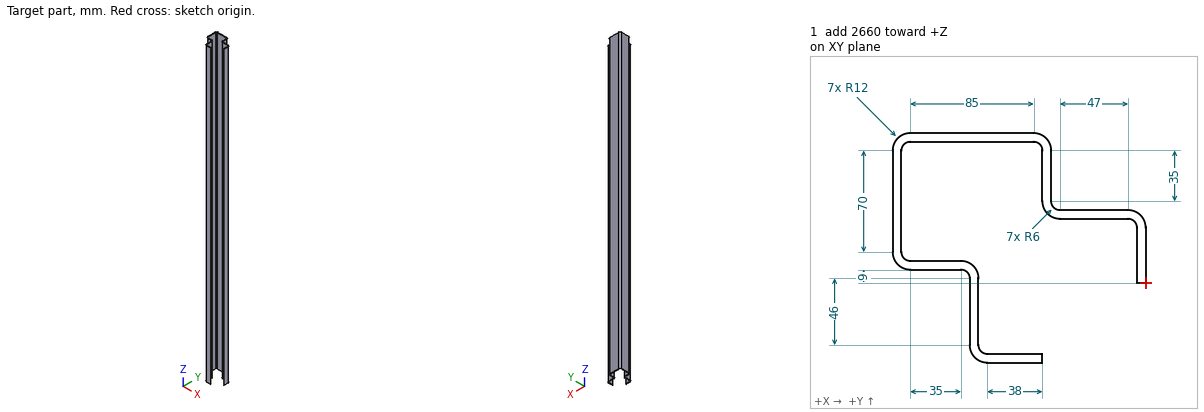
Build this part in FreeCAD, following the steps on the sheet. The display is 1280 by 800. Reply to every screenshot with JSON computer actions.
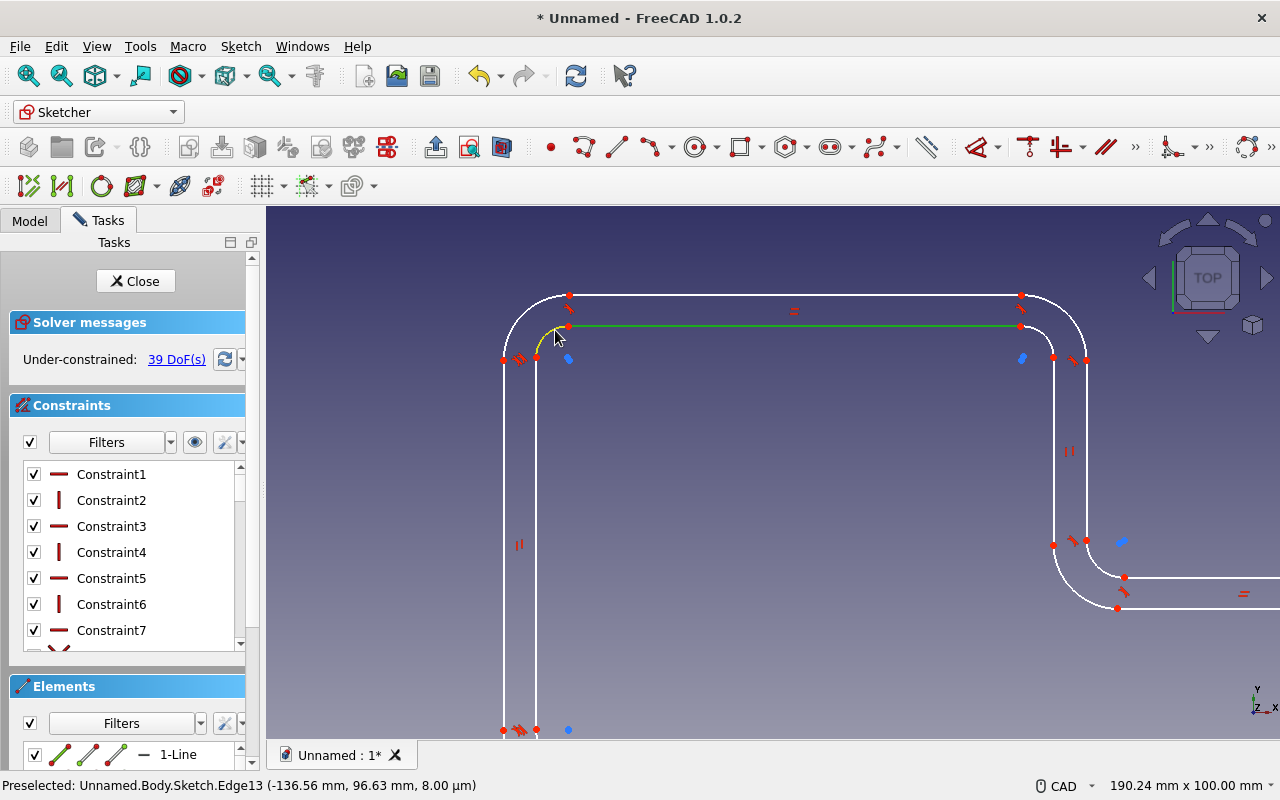
{"action": "left_click", "coordinate": [554, 329]}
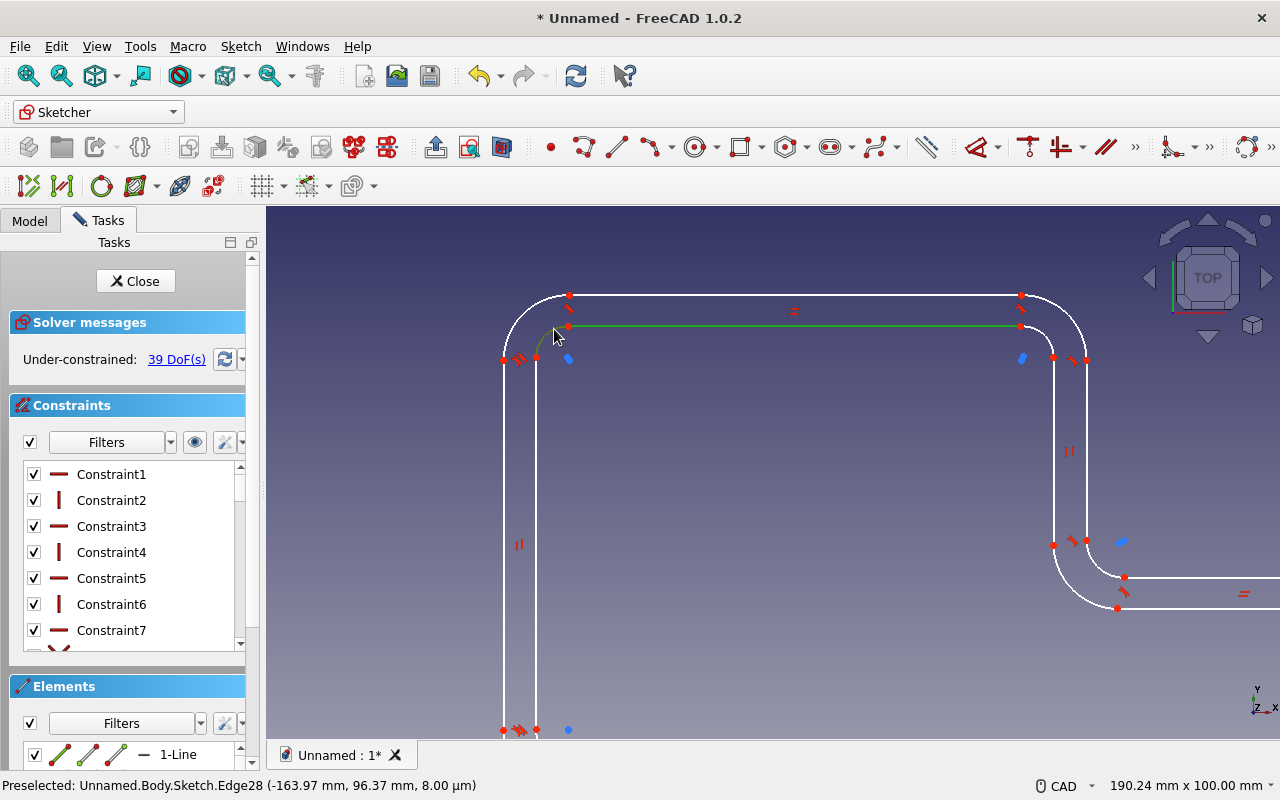
{"action": "key", "text": "t"}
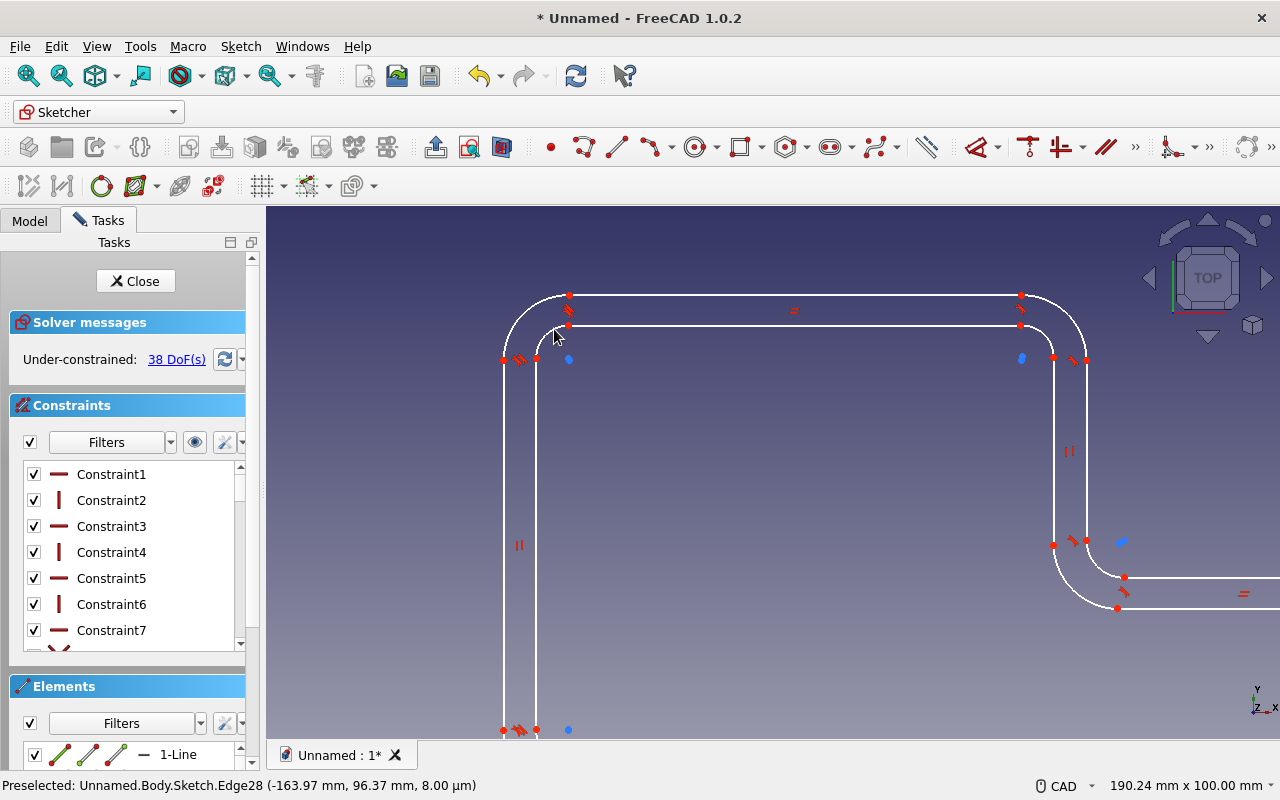
{"action": "left_click", "coordinate": [704, 326]}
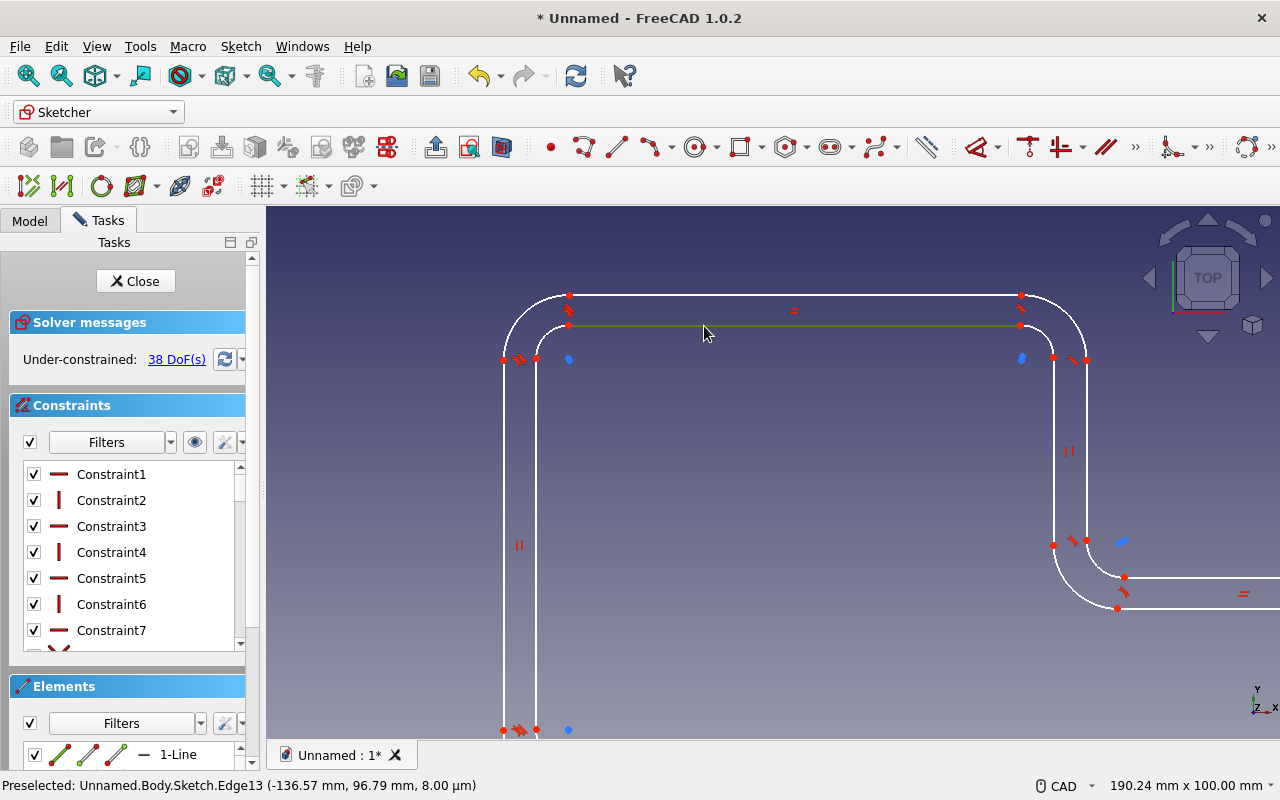
{"action": "left_click", "coordinate": [1050, 343]}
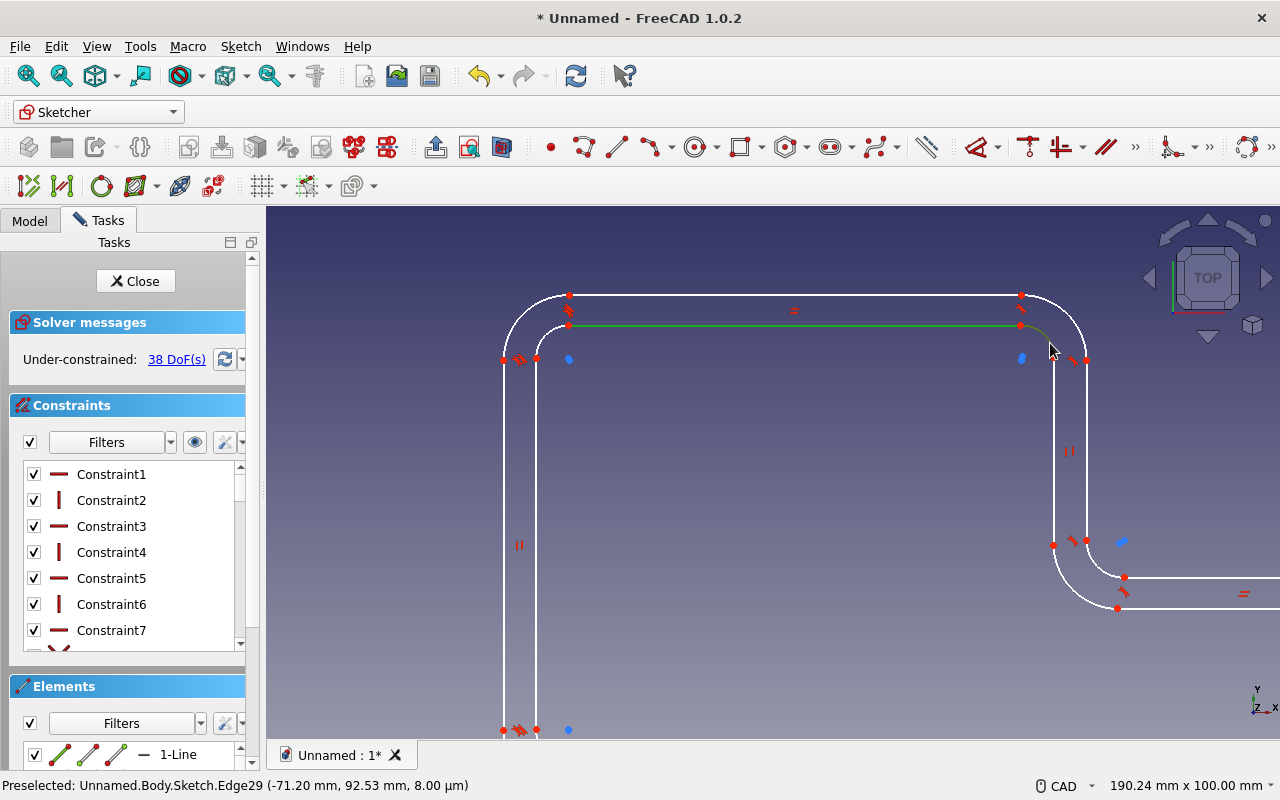
{"action": "key", "text": "t"}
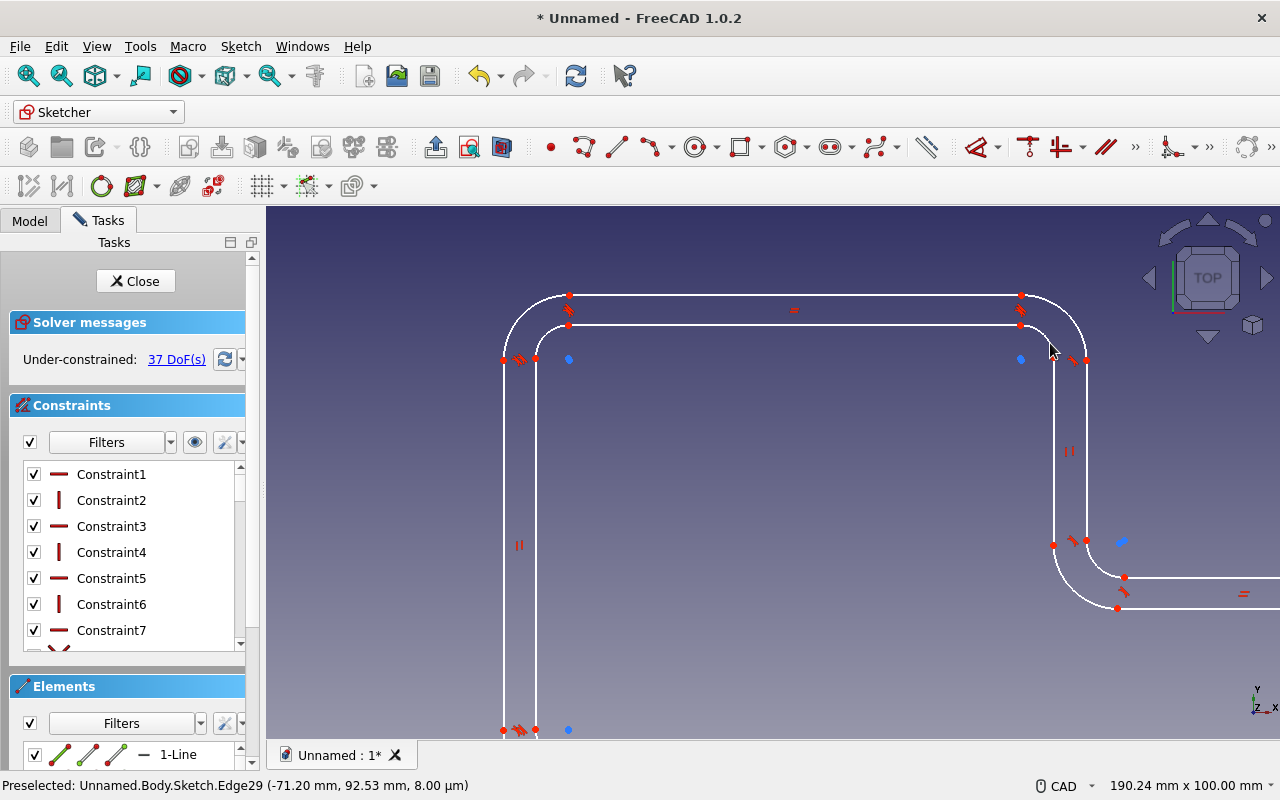
{"action": "left_click", "coordinate": [1054, 414]}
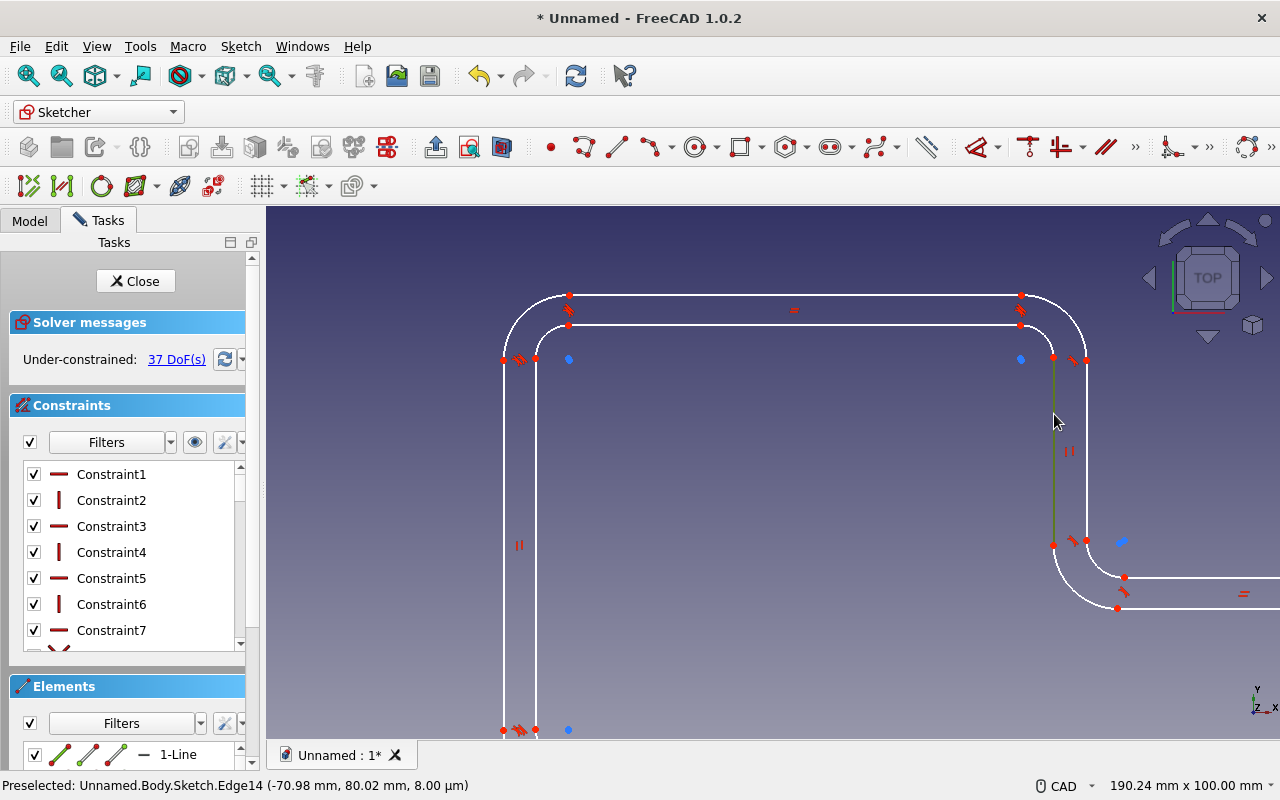
{"action": "left_click", "coordinate": [1050, 343]}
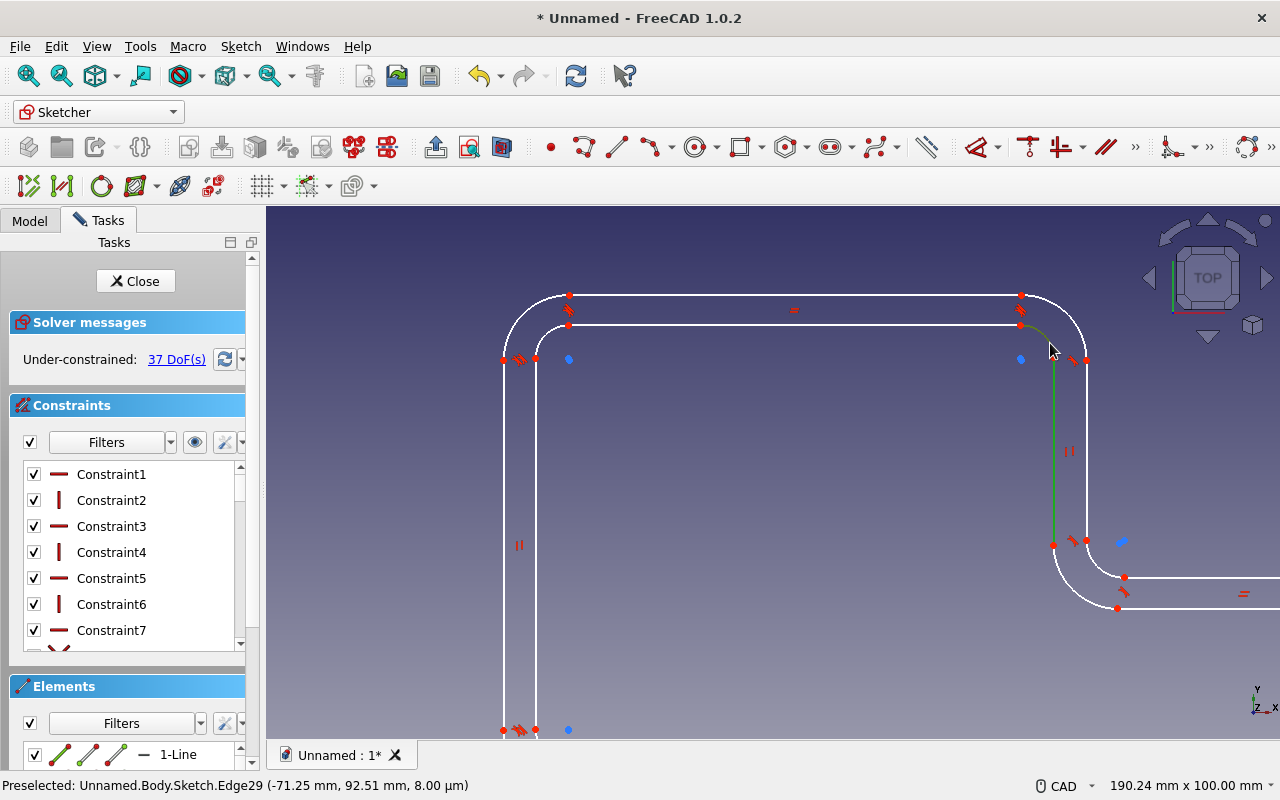
{"action": "key", "text": "t"}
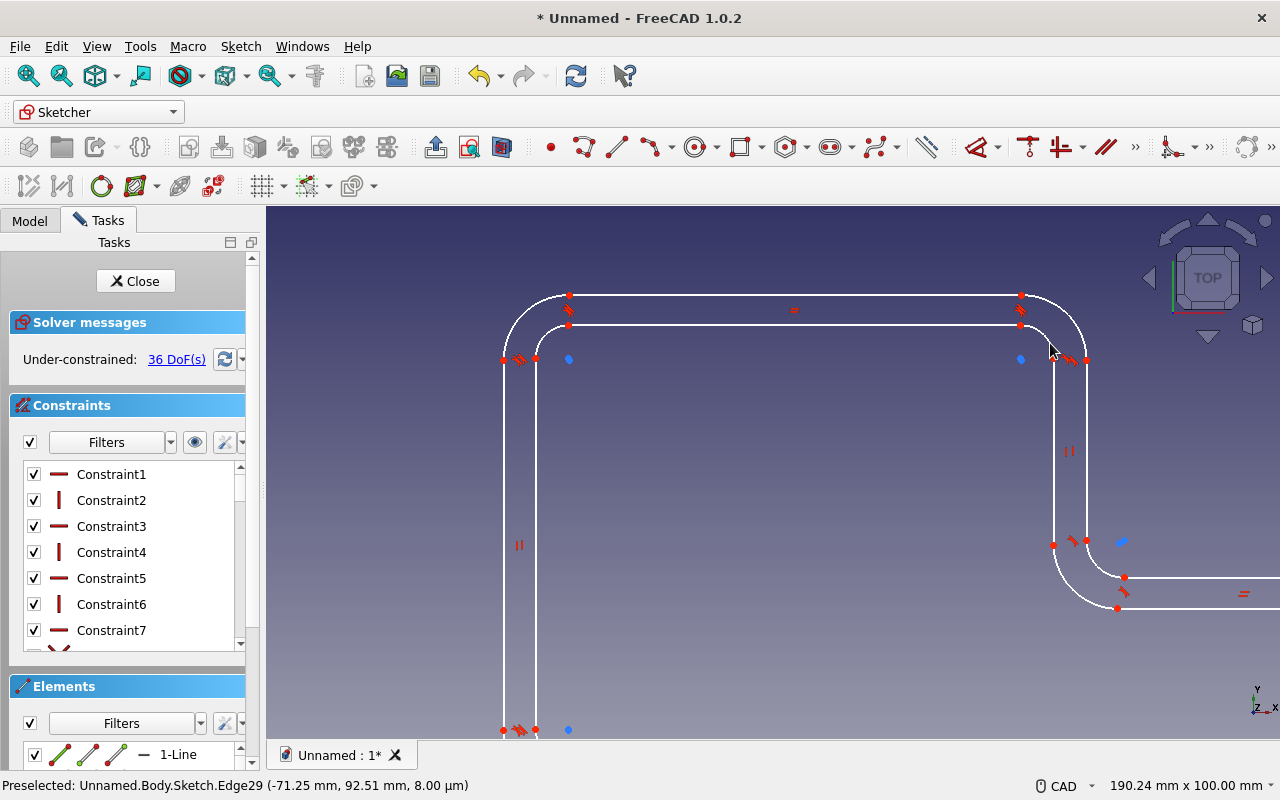
{"action": "left_click", "coordinate": [1054, 414]}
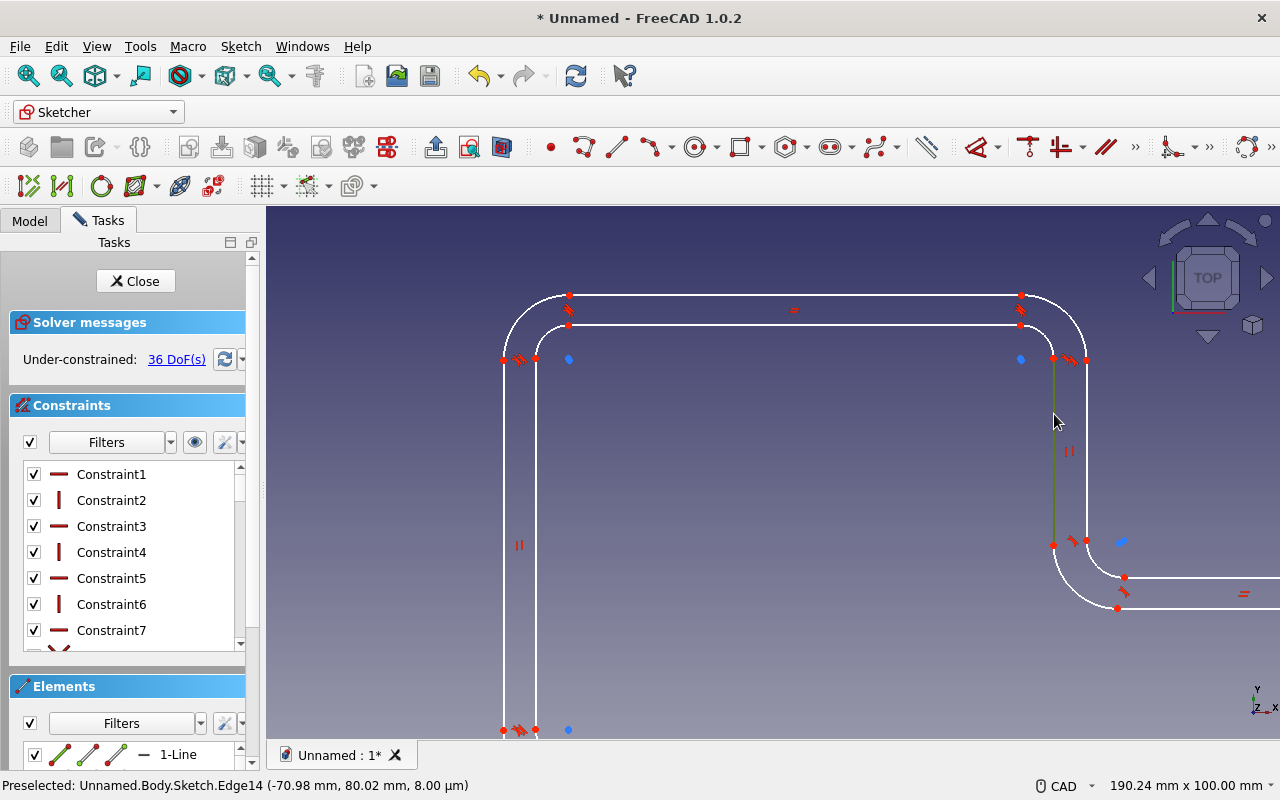
{"action": "left_click", "coordinate": [1061, 574]}